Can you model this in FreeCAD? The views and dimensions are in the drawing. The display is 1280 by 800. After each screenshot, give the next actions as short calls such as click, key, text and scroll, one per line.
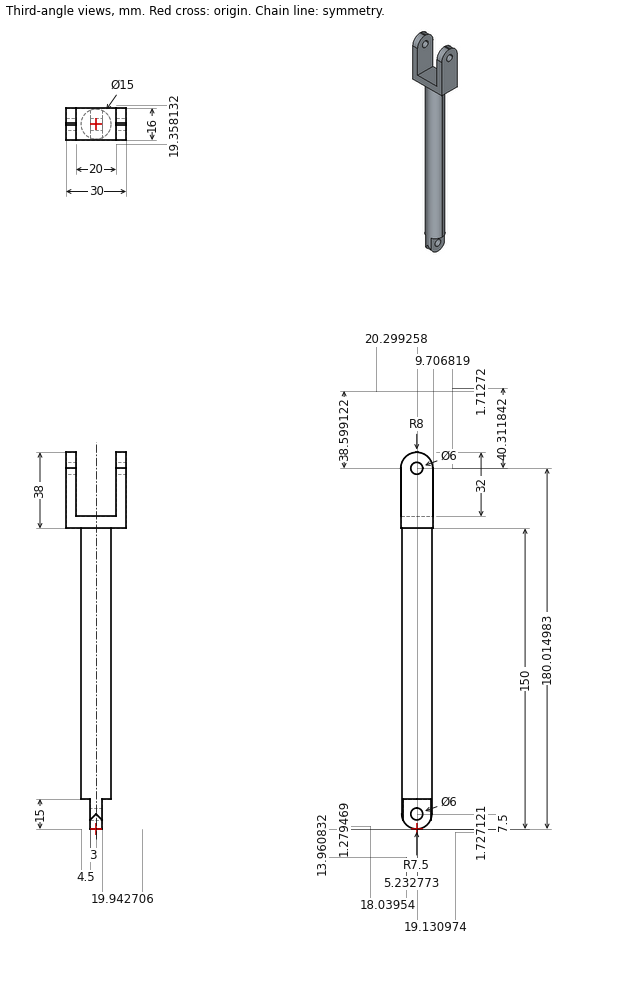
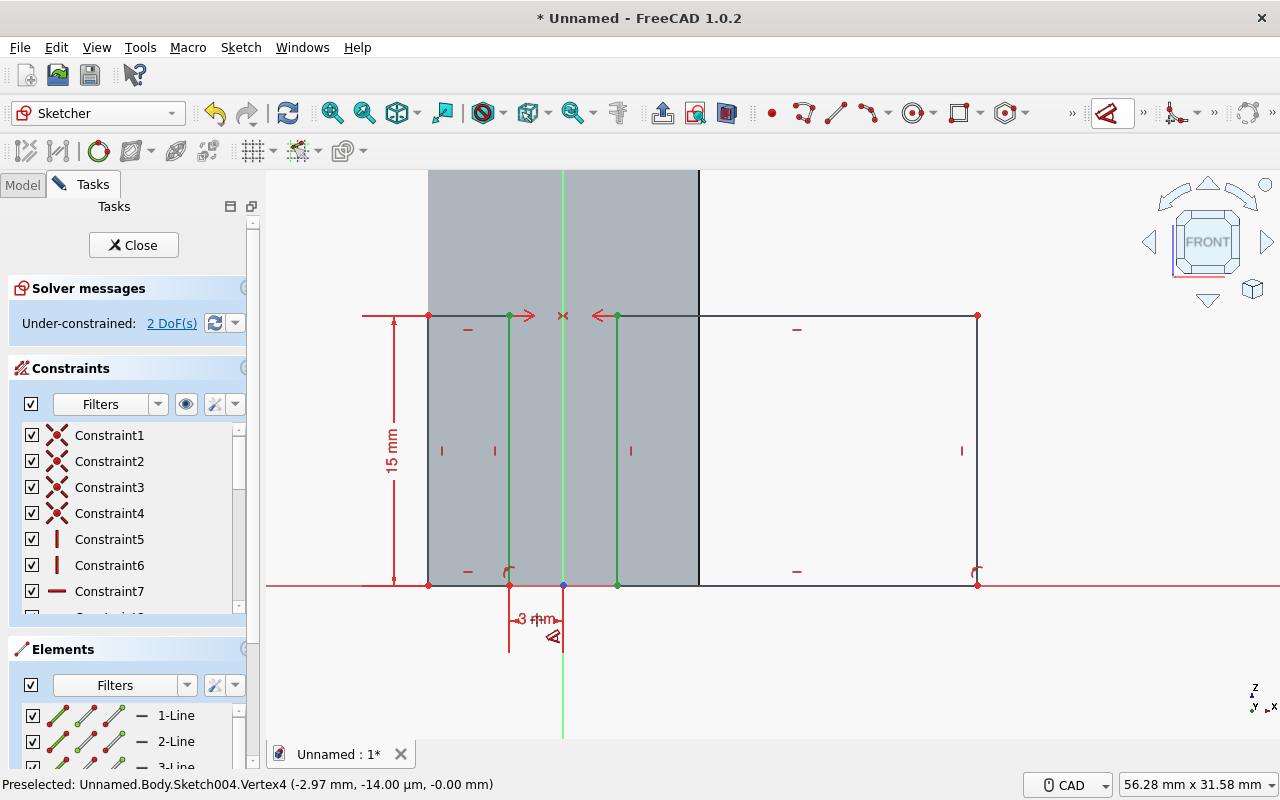
click(452, 586)
click(450, 620)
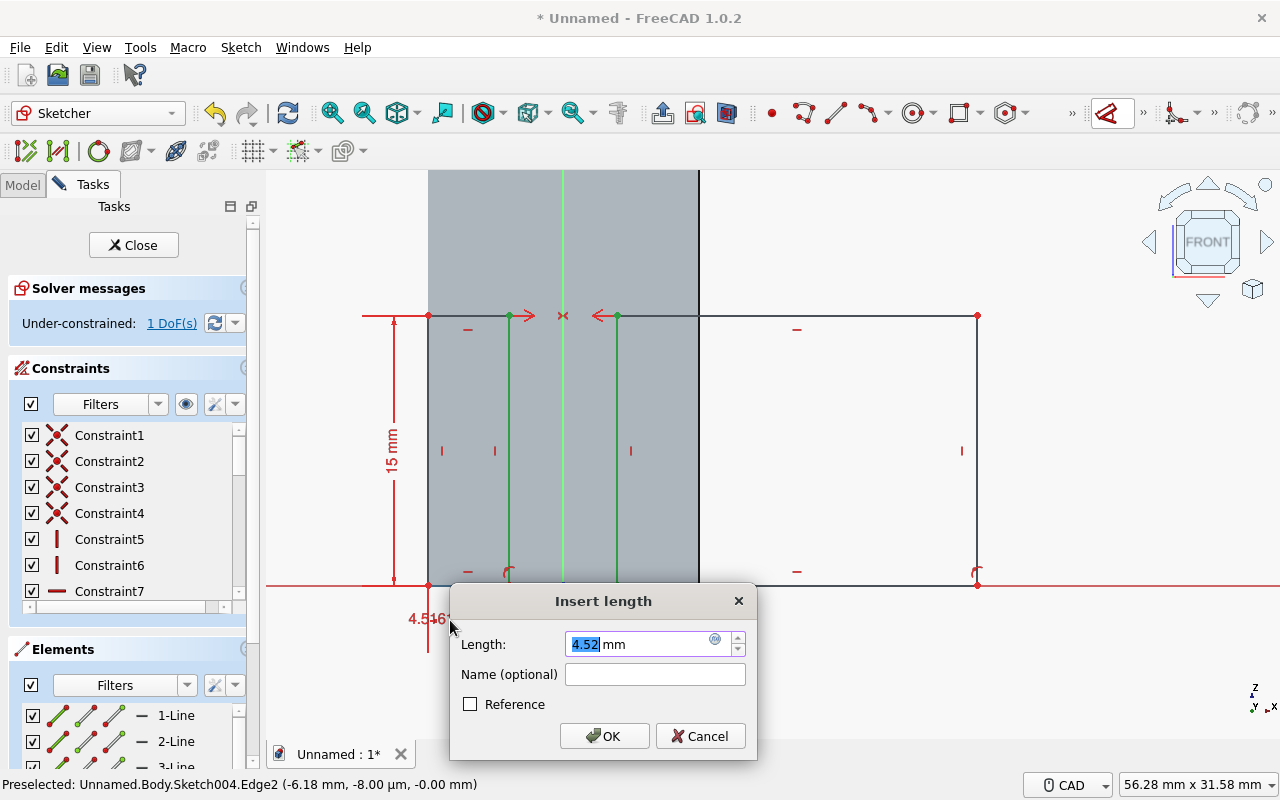
text(4.5)
key(Return)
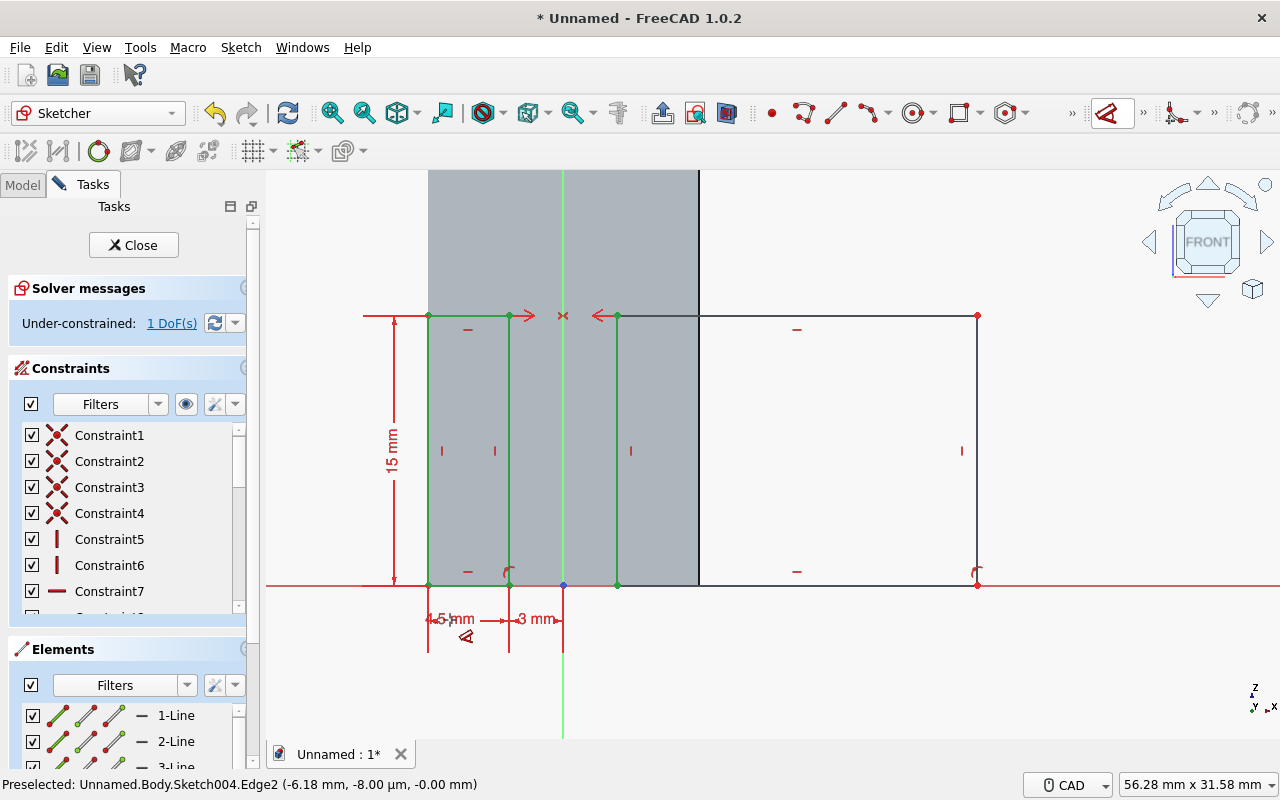
click(725, 586)
click(797, 620)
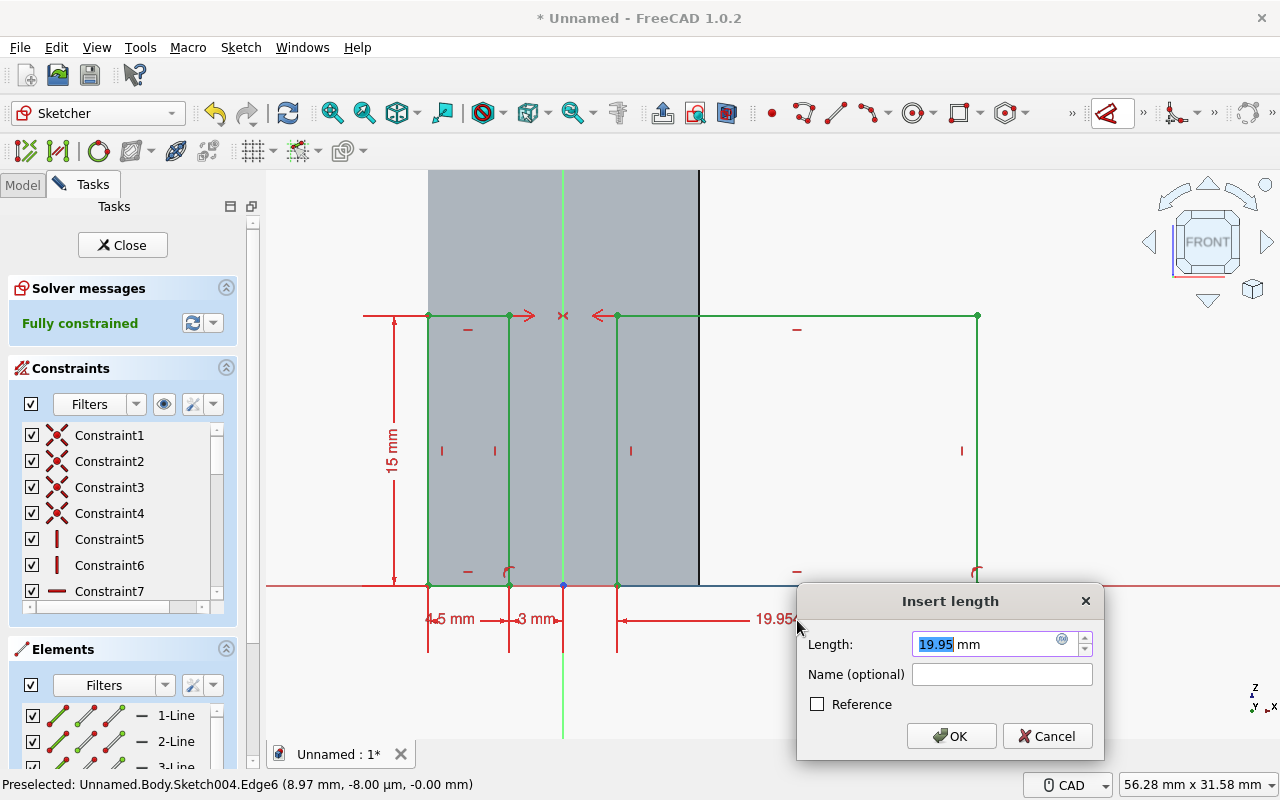
text(19.942706)
key(Return)
key(Escape)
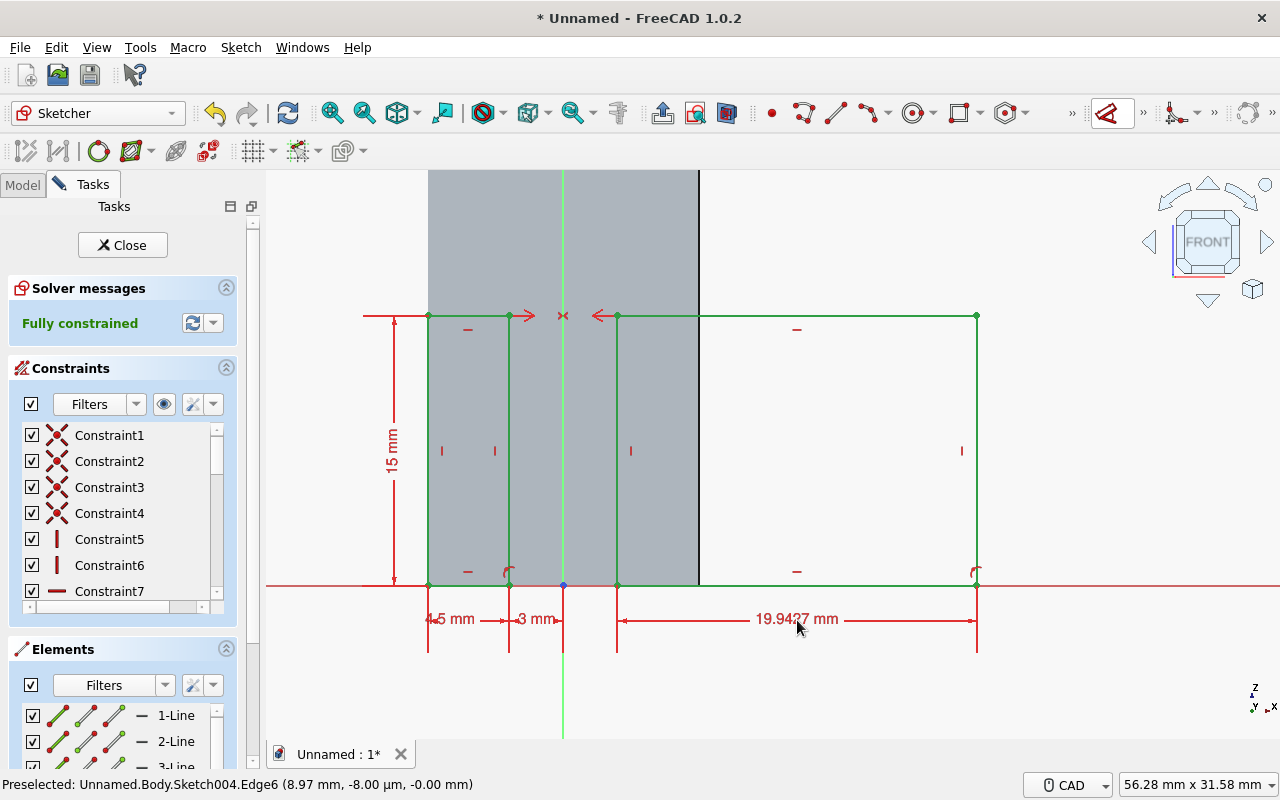
click(123, 245)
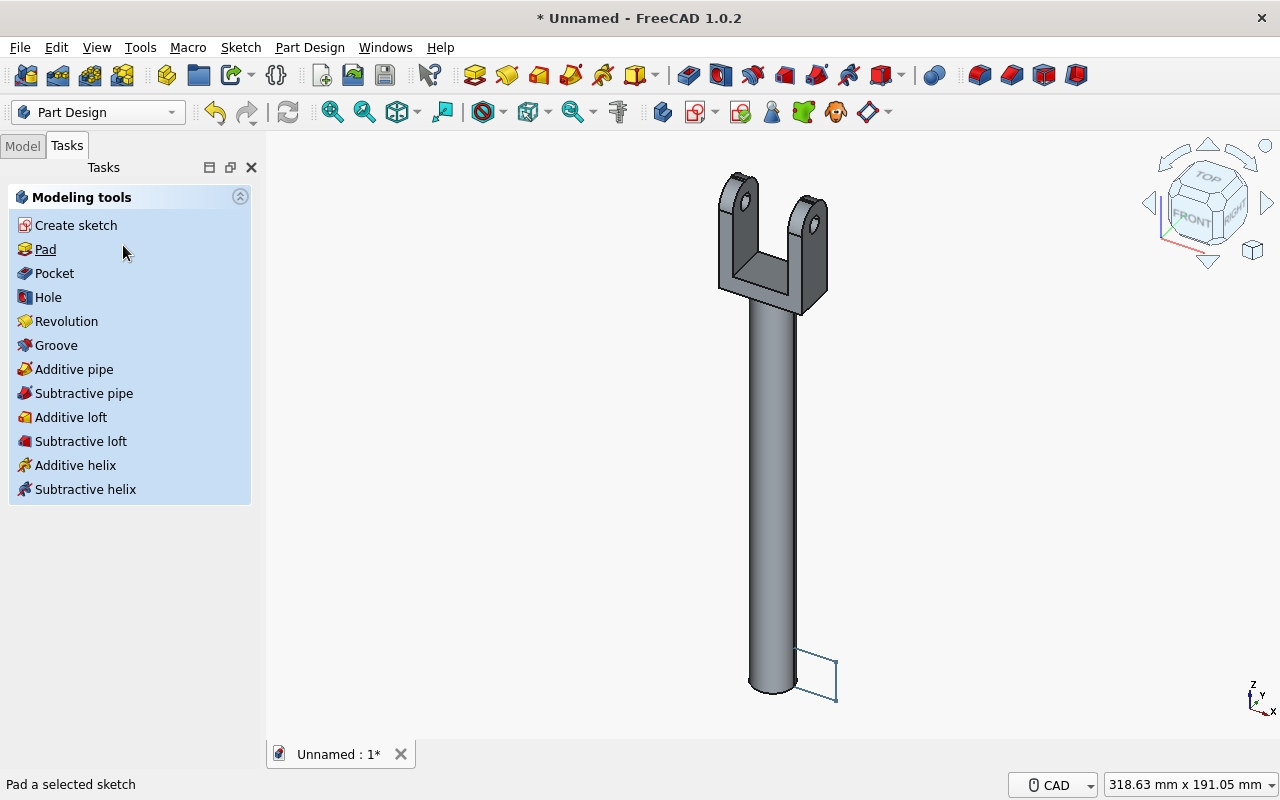
click(690, 76)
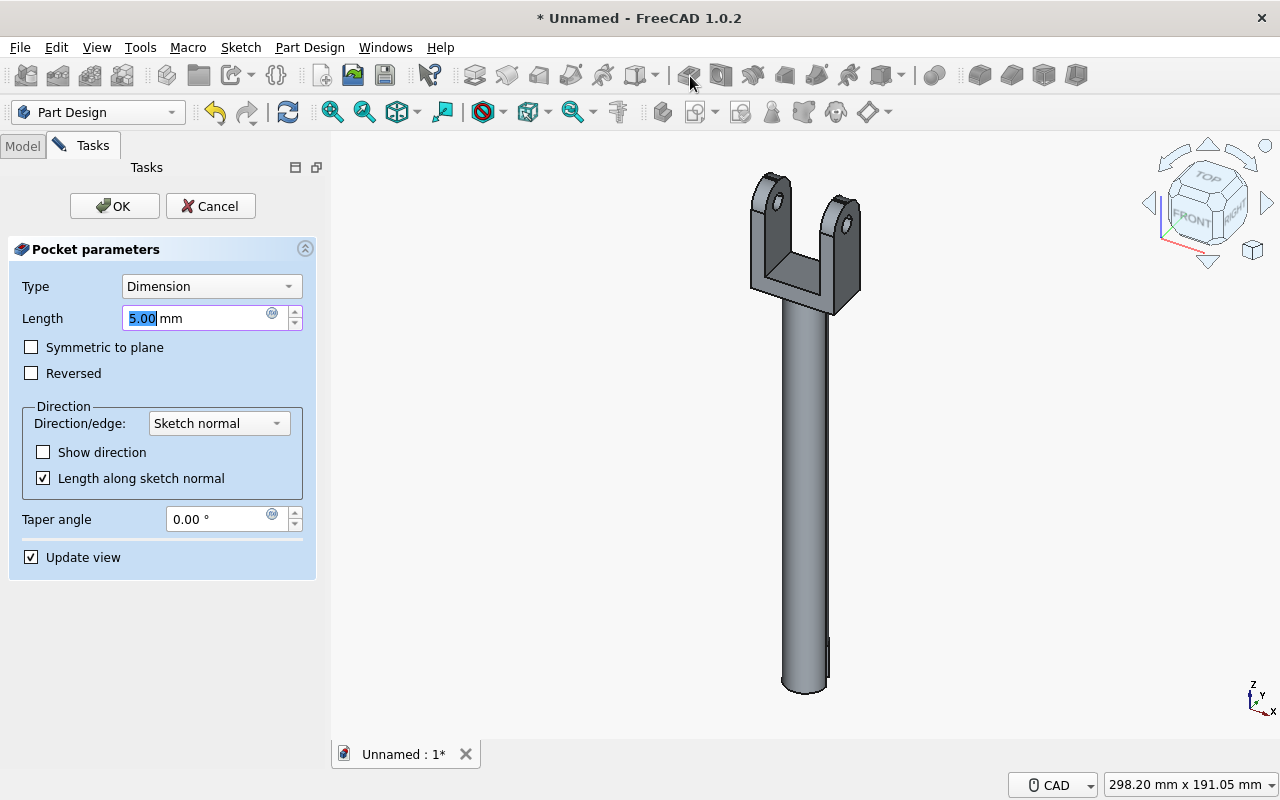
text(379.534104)
key(Tab)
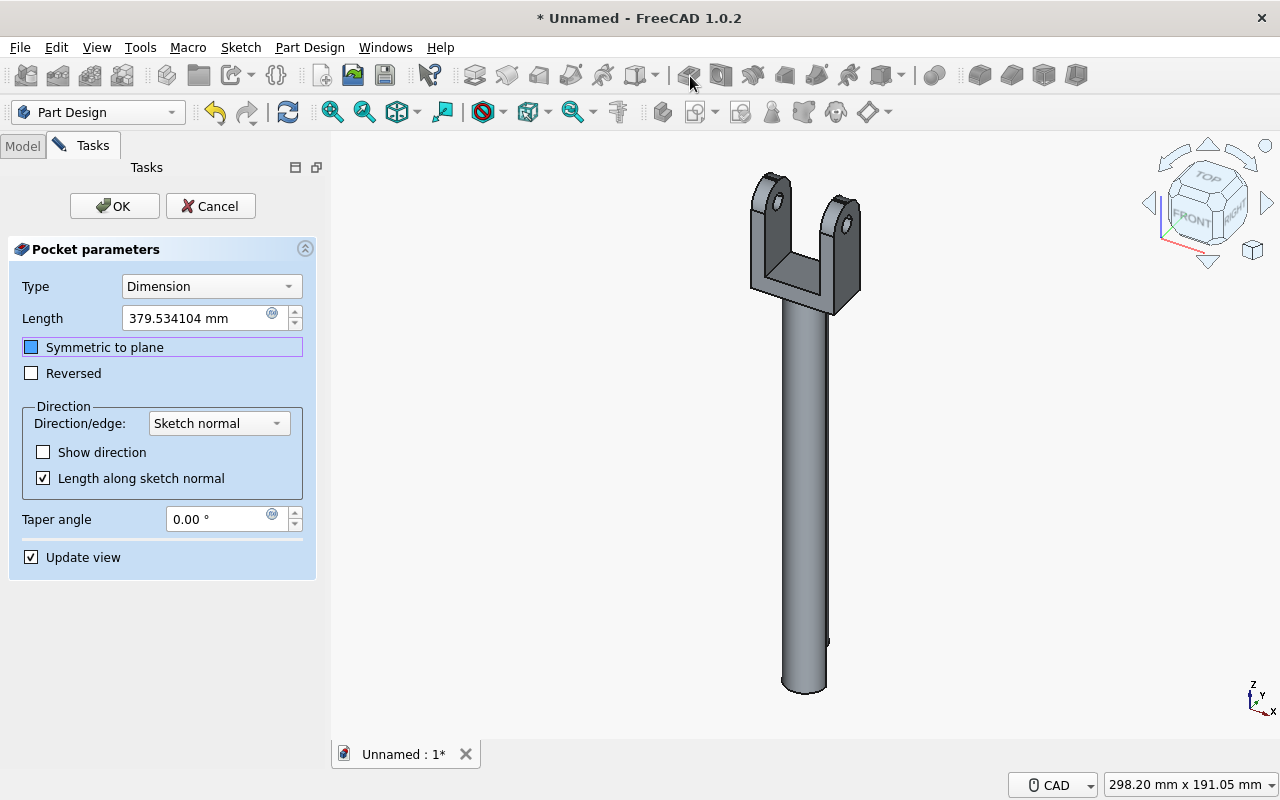
click(30, 347)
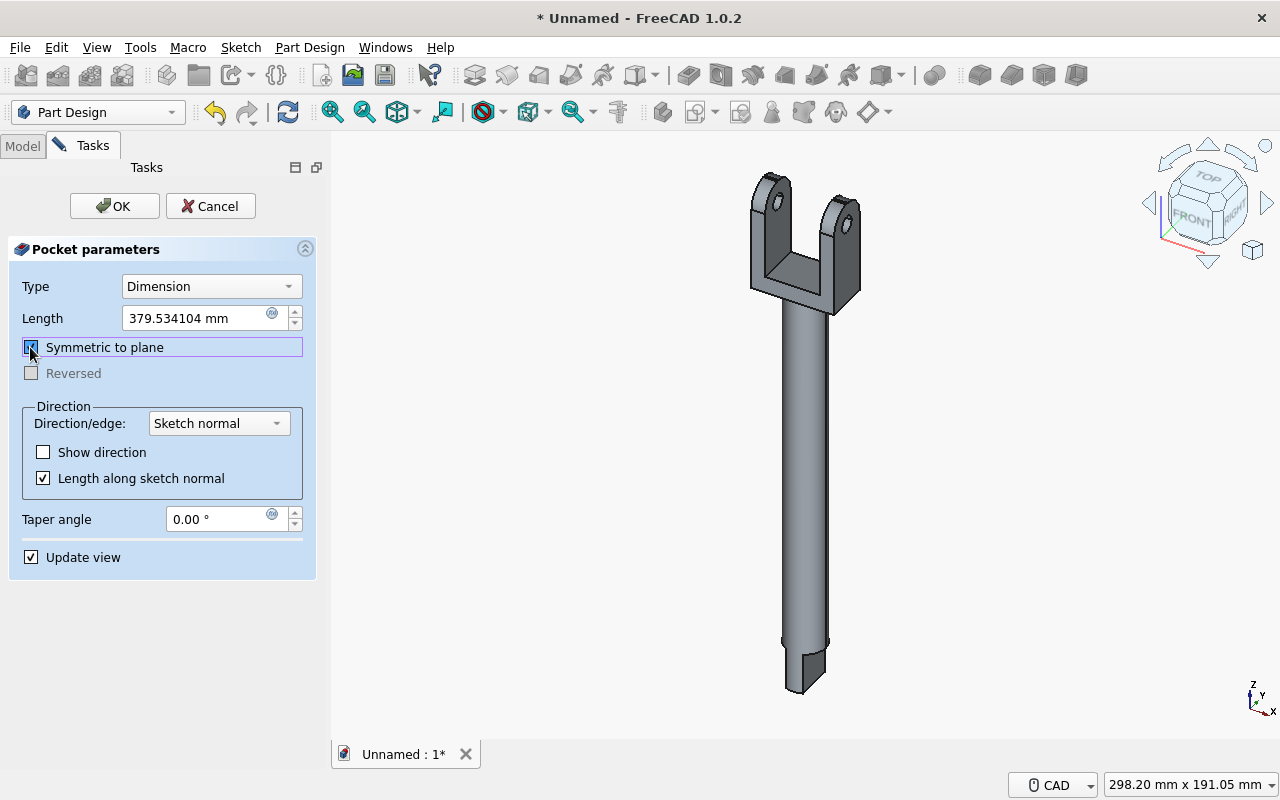
click(115, 206)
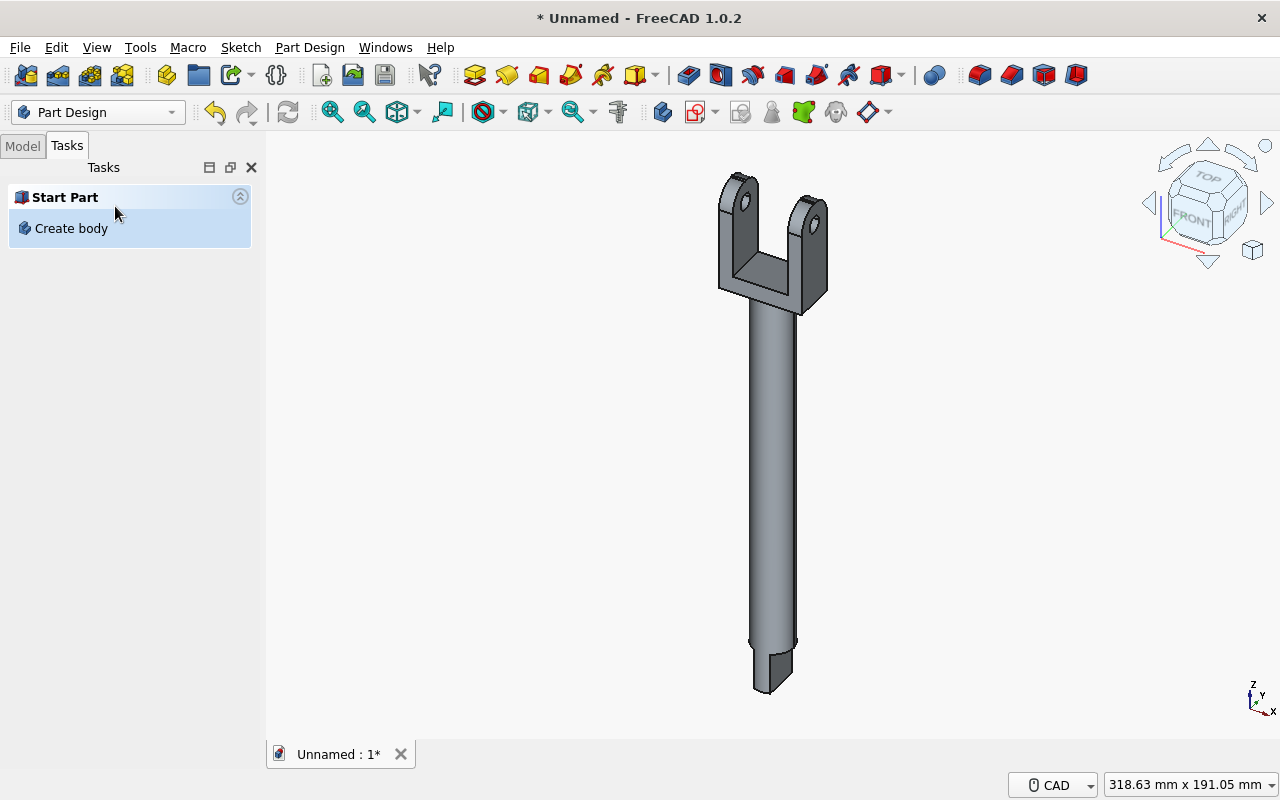
key(6)